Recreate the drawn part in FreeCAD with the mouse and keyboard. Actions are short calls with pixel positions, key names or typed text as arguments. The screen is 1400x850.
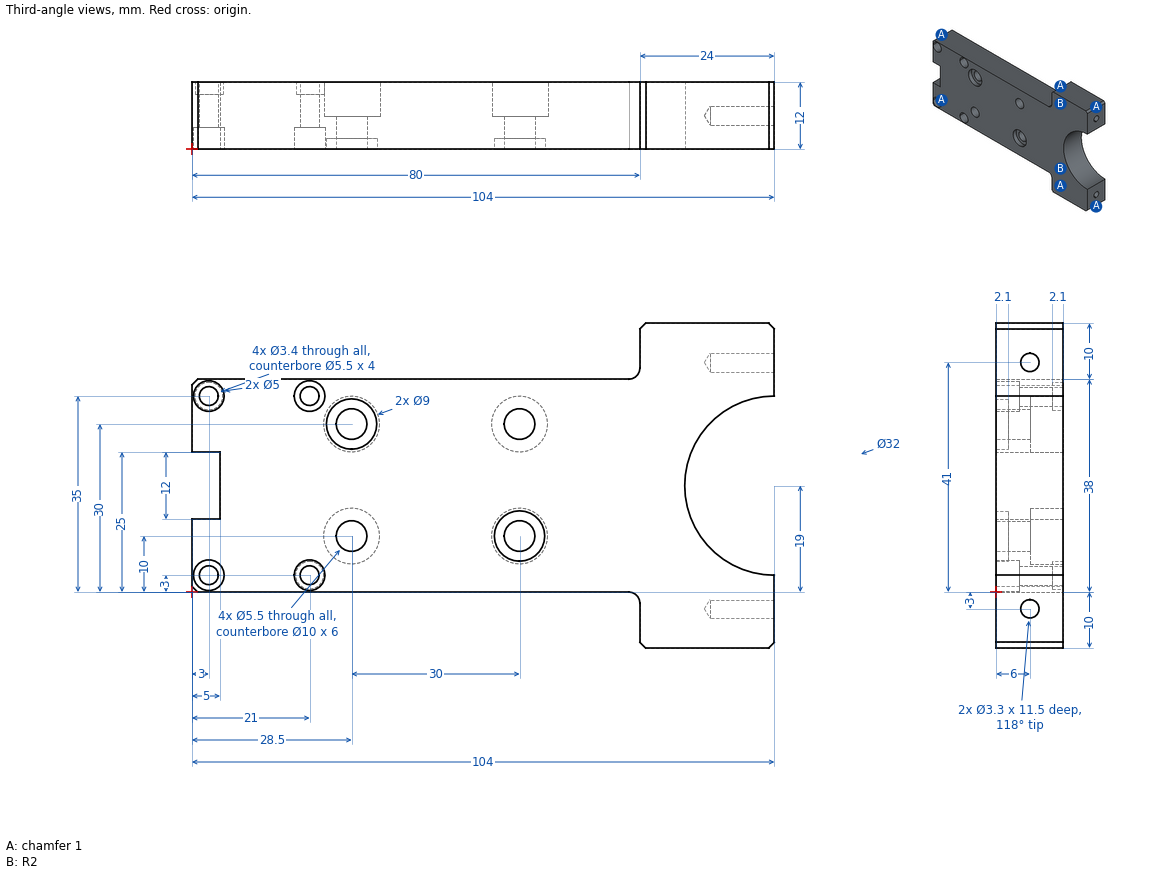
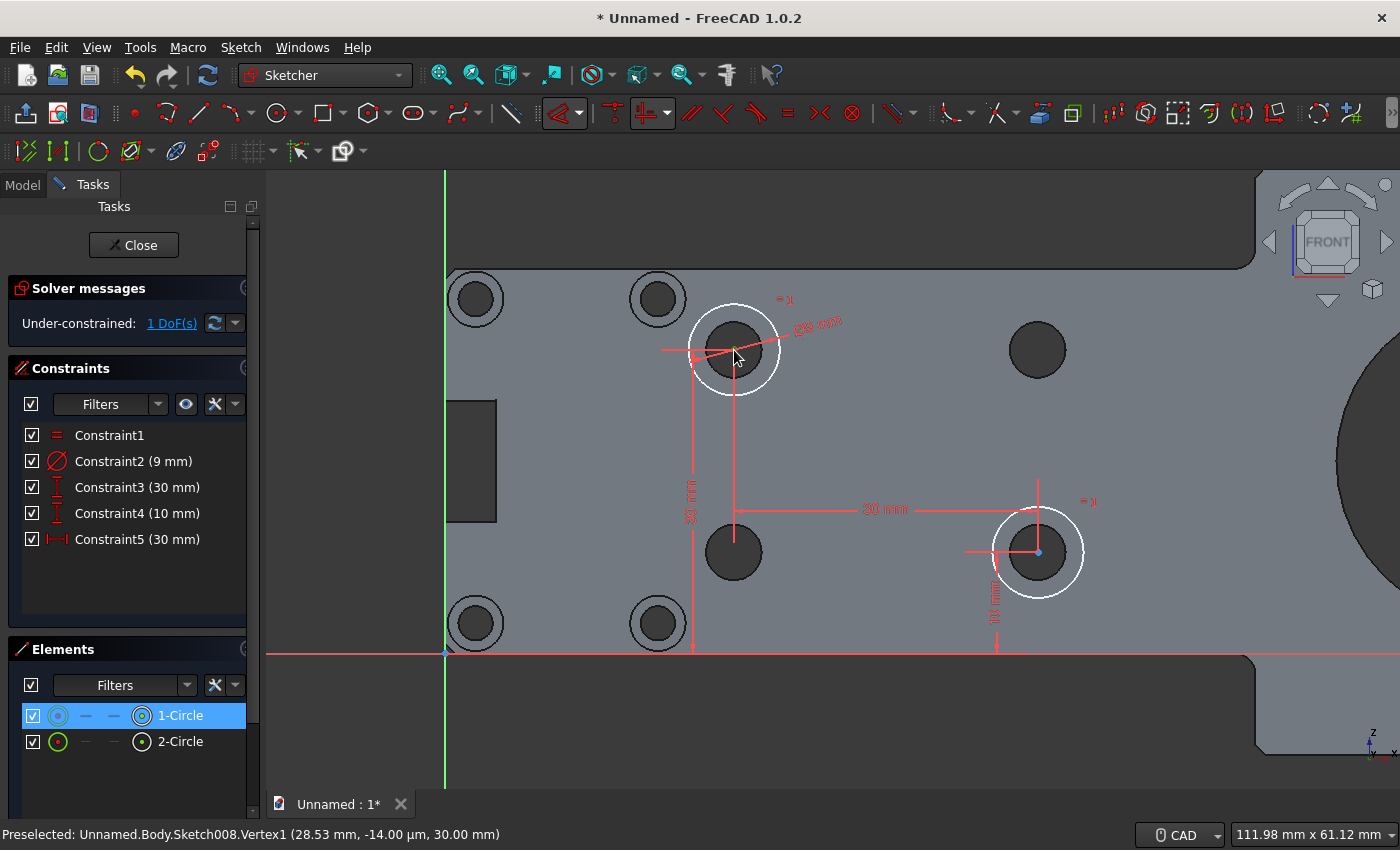
click(582, 114)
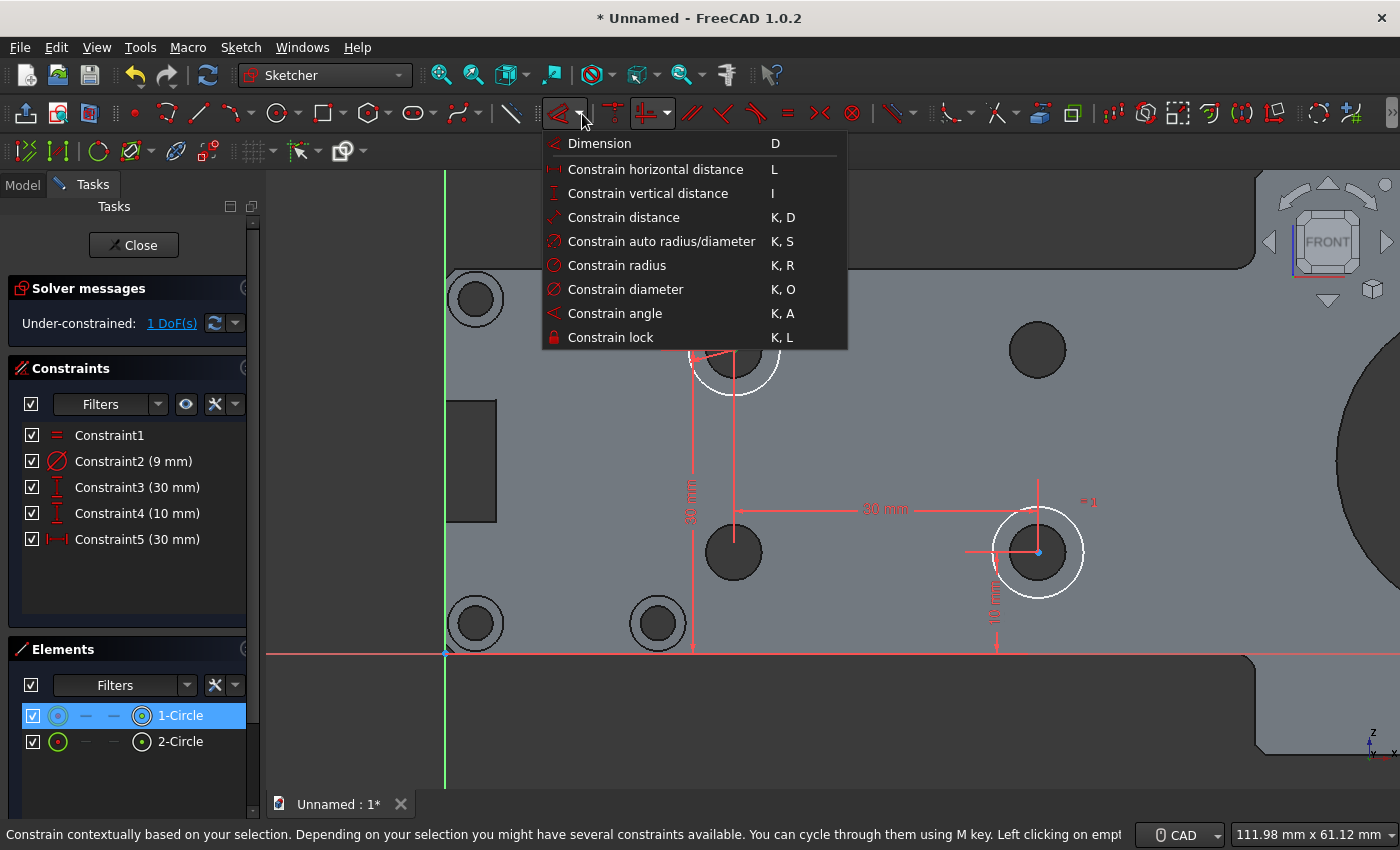
click(695, 169)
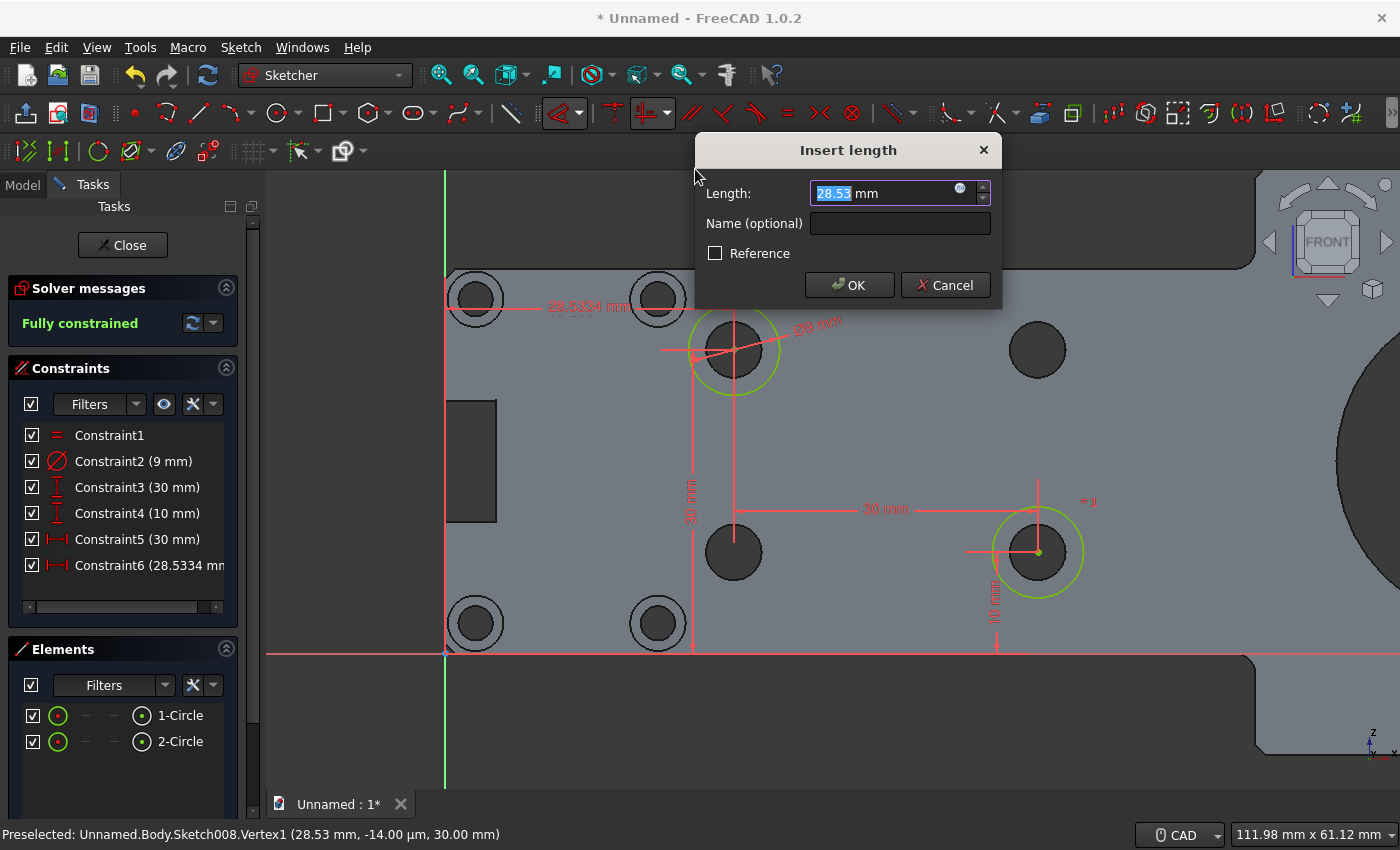
text(28.5)
key(Return)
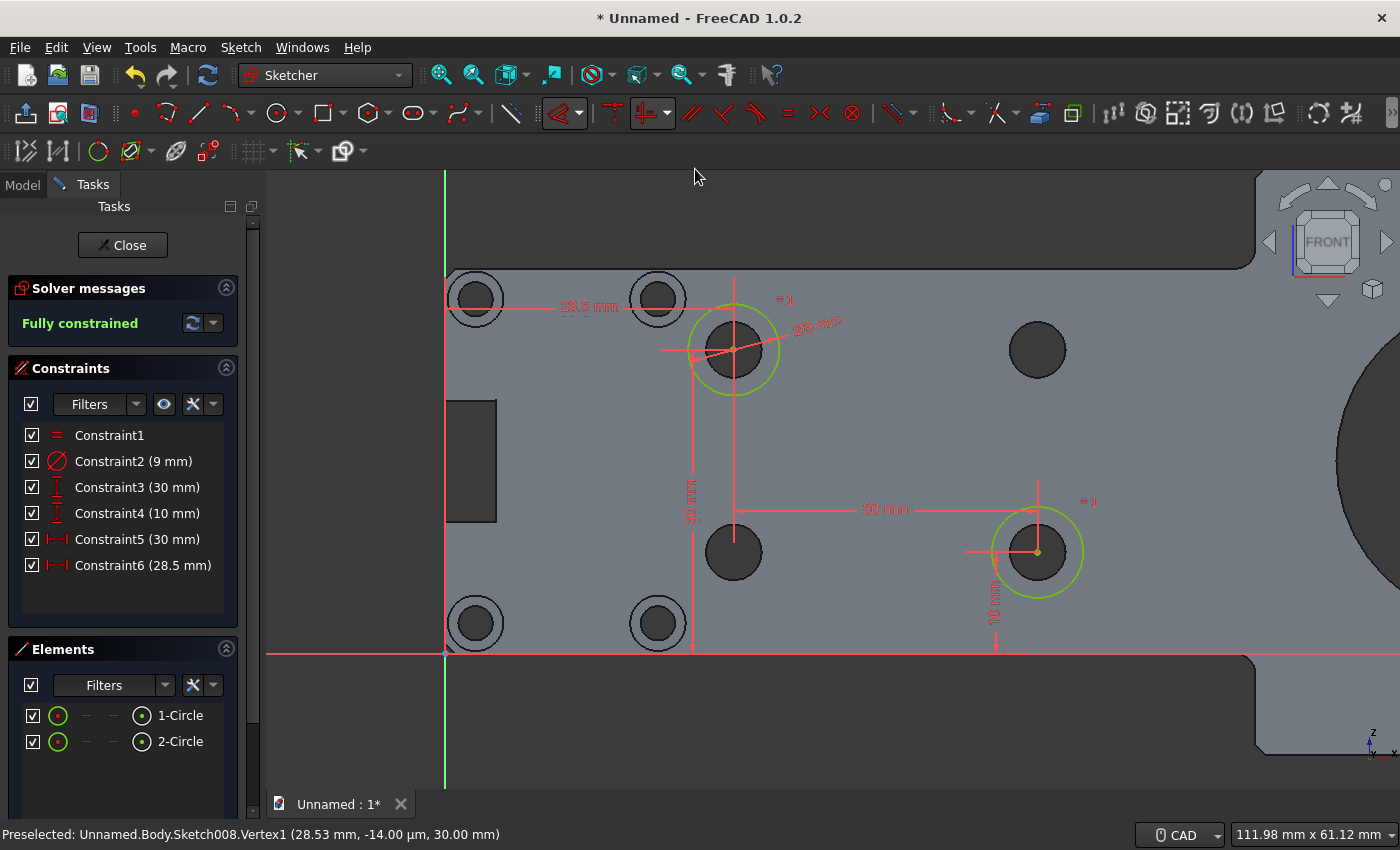
click(123, 245)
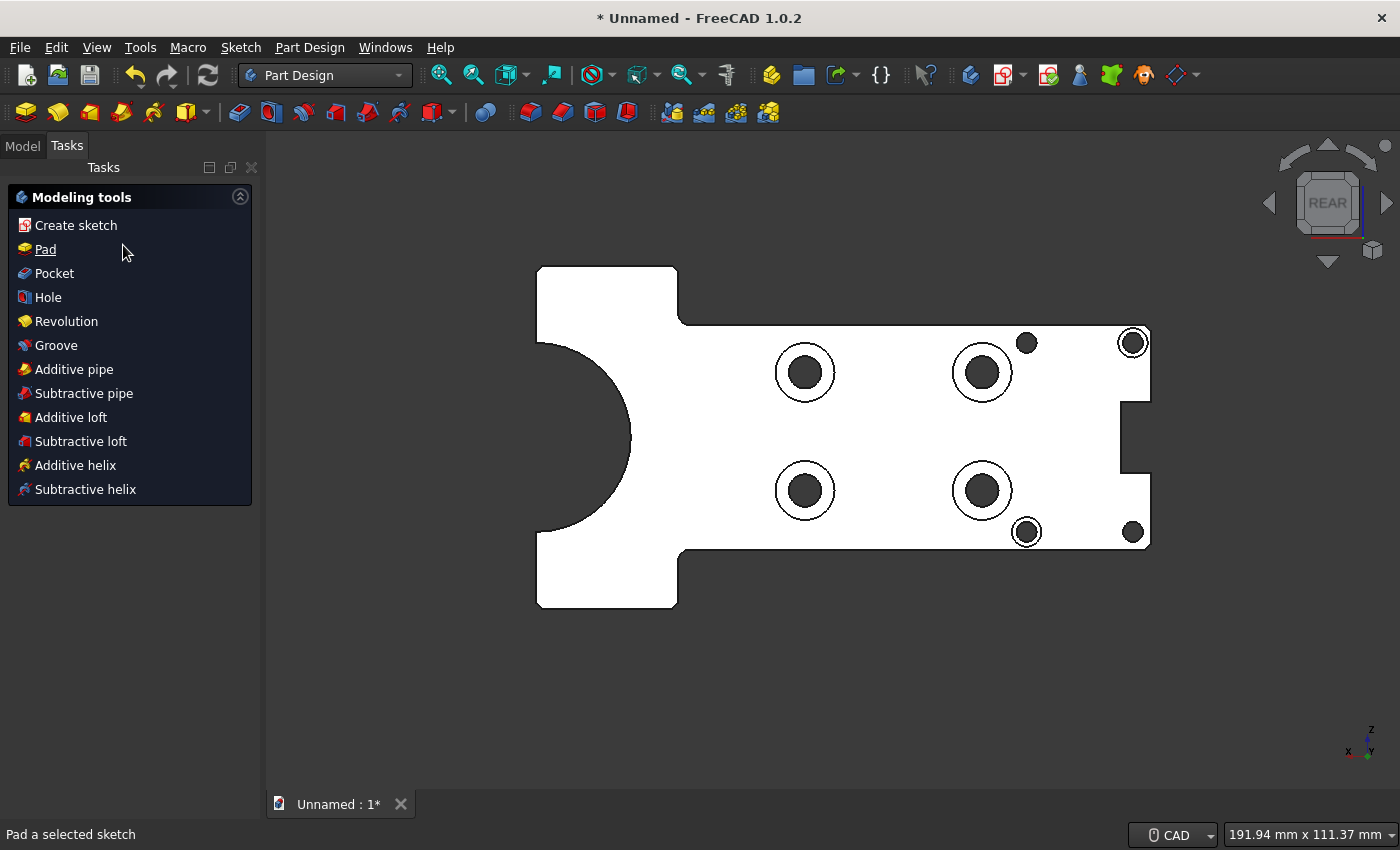
click(240, 112)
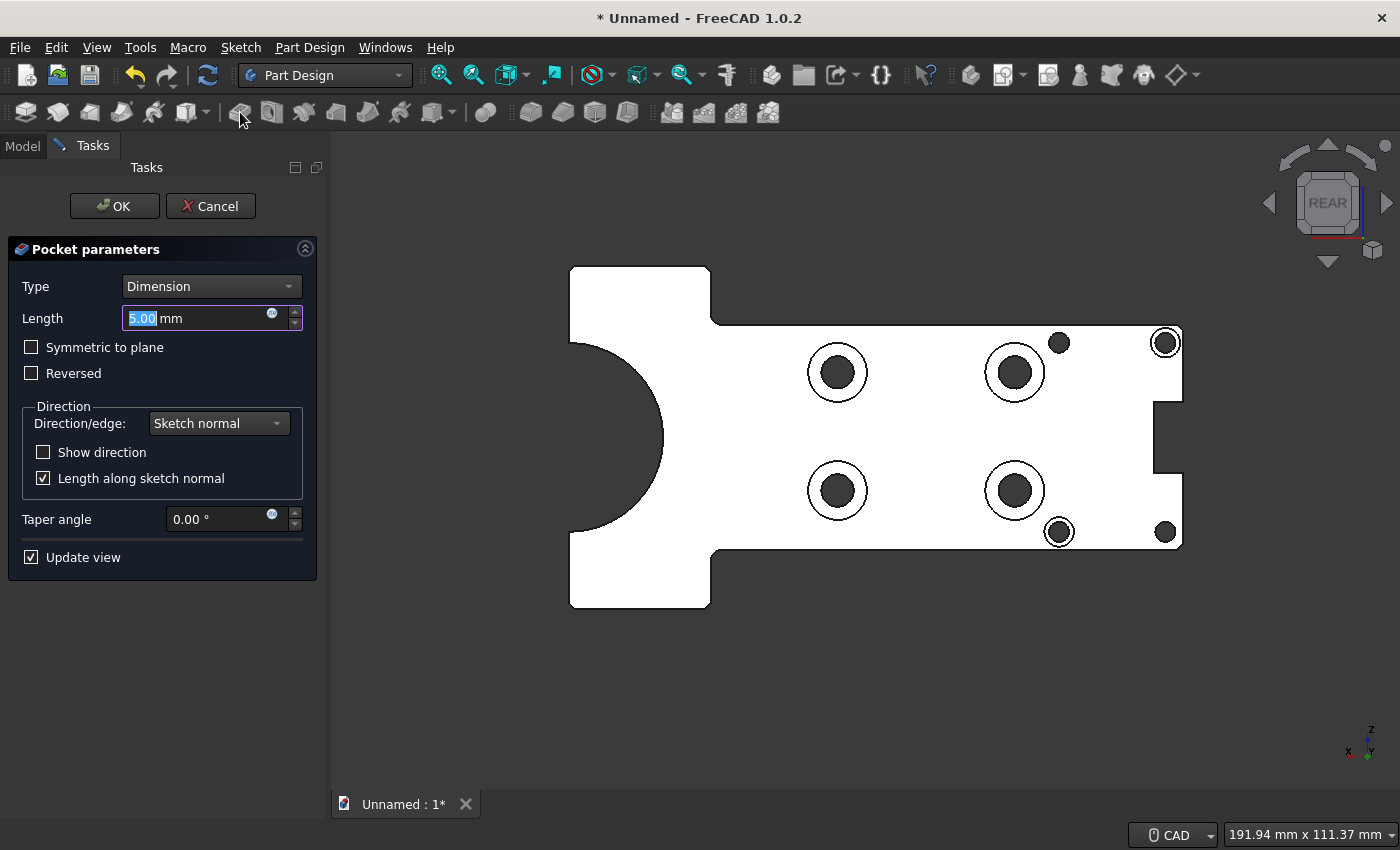
text(2.1)
key(Tab)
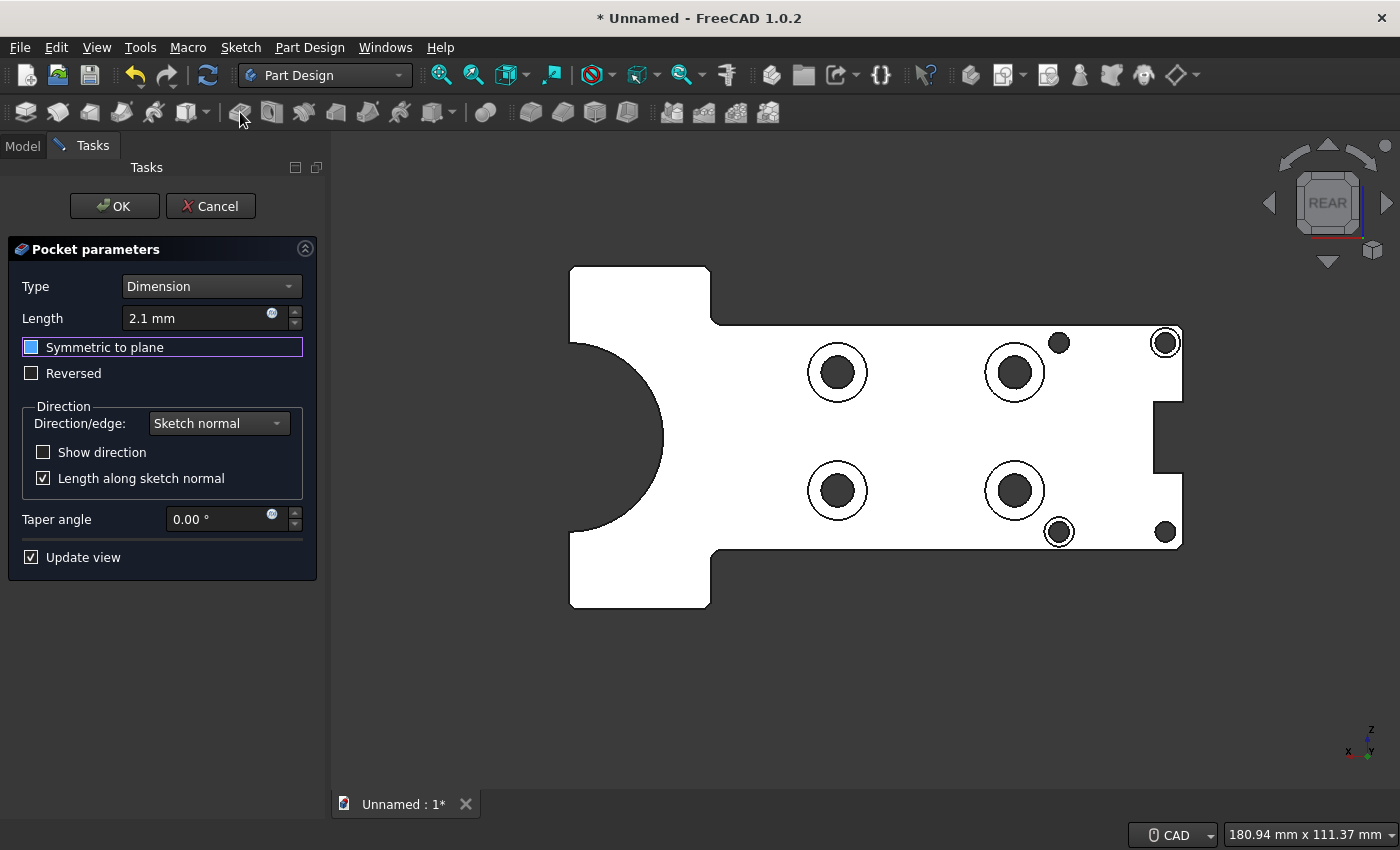
click(115, 206)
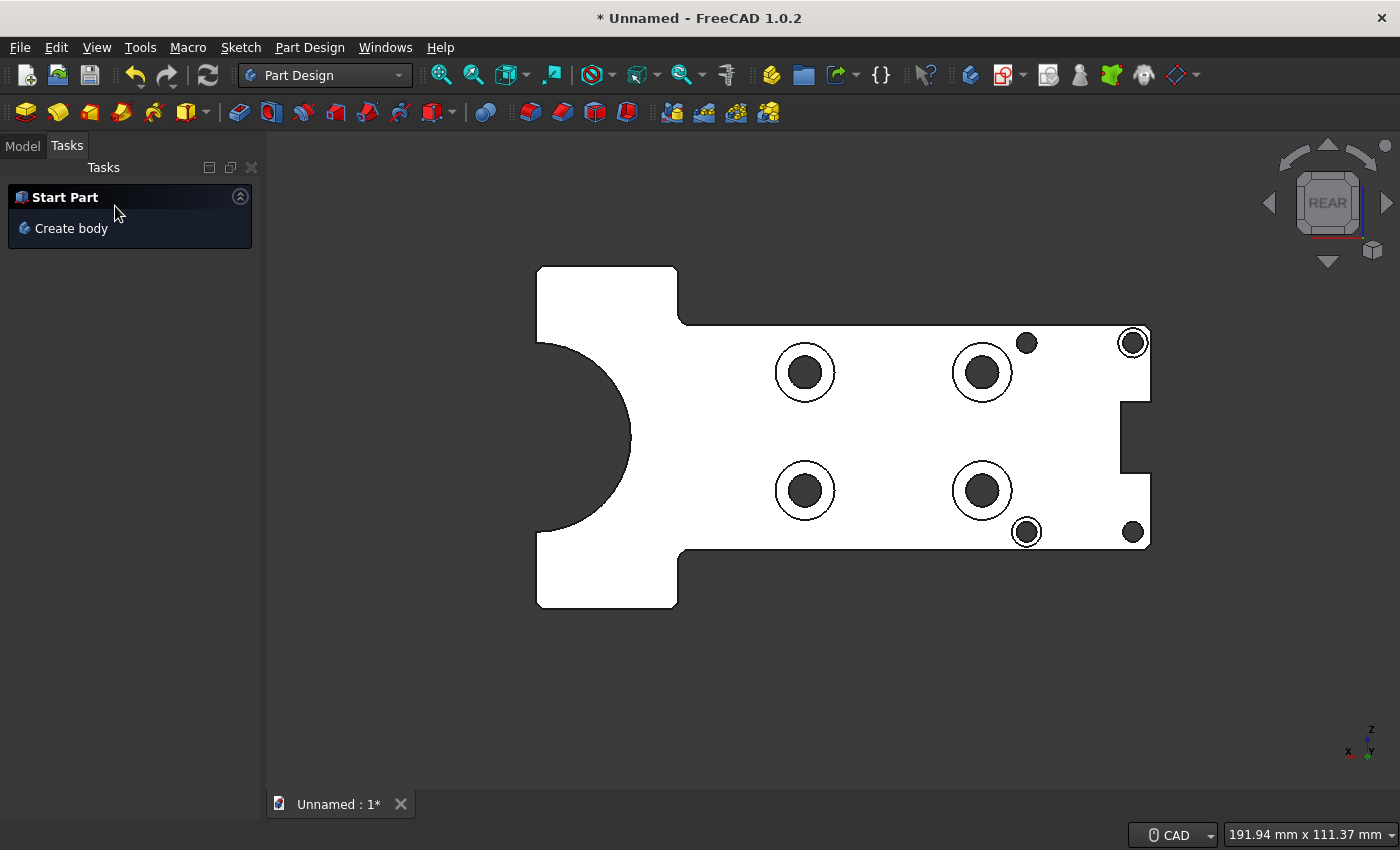
key(0)